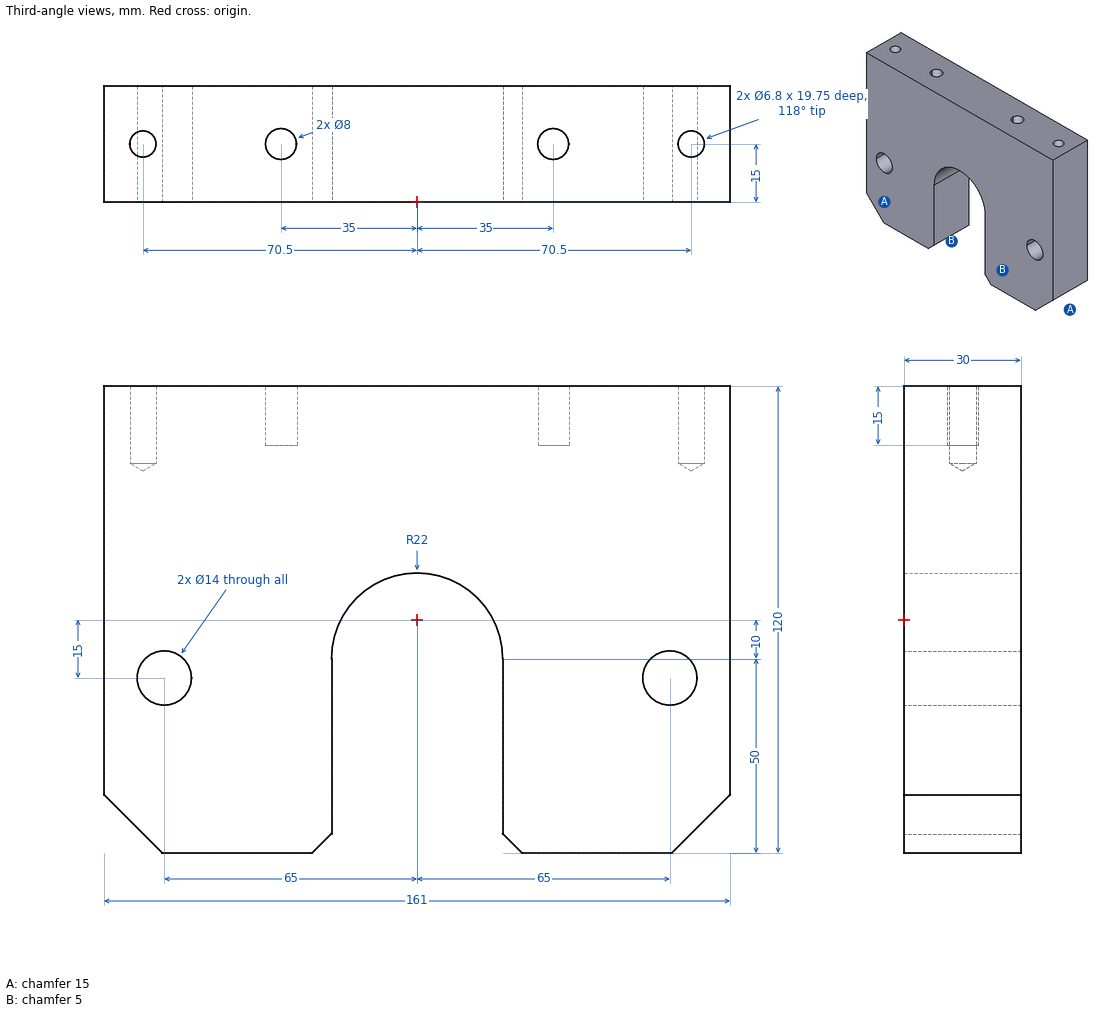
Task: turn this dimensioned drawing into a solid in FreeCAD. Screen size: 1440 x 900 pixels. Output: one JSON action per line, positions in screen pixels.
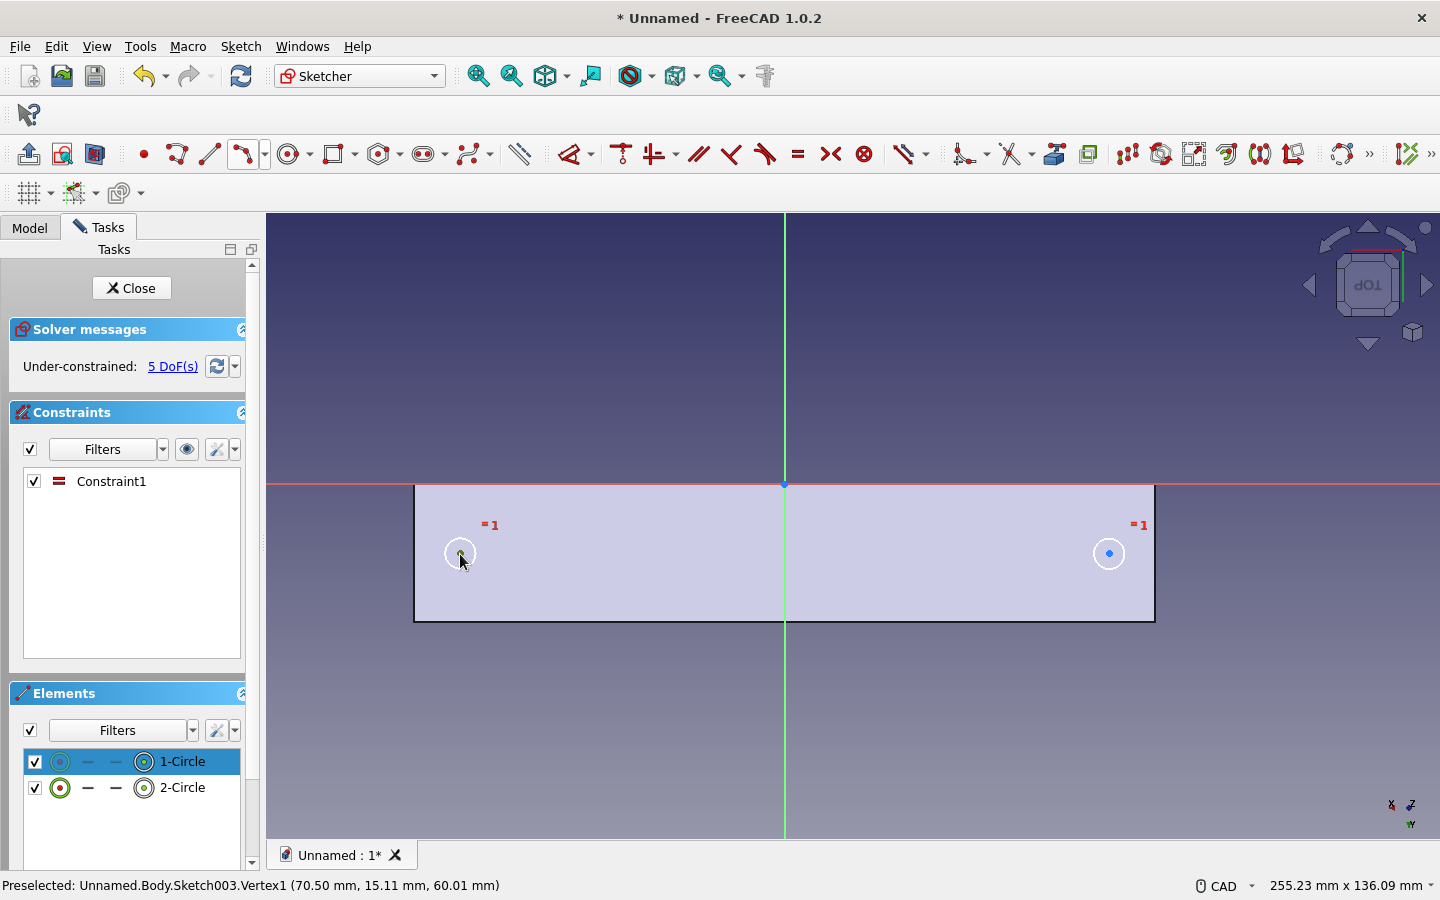
{"action": "left_click", "coordinate": [1109, 554]}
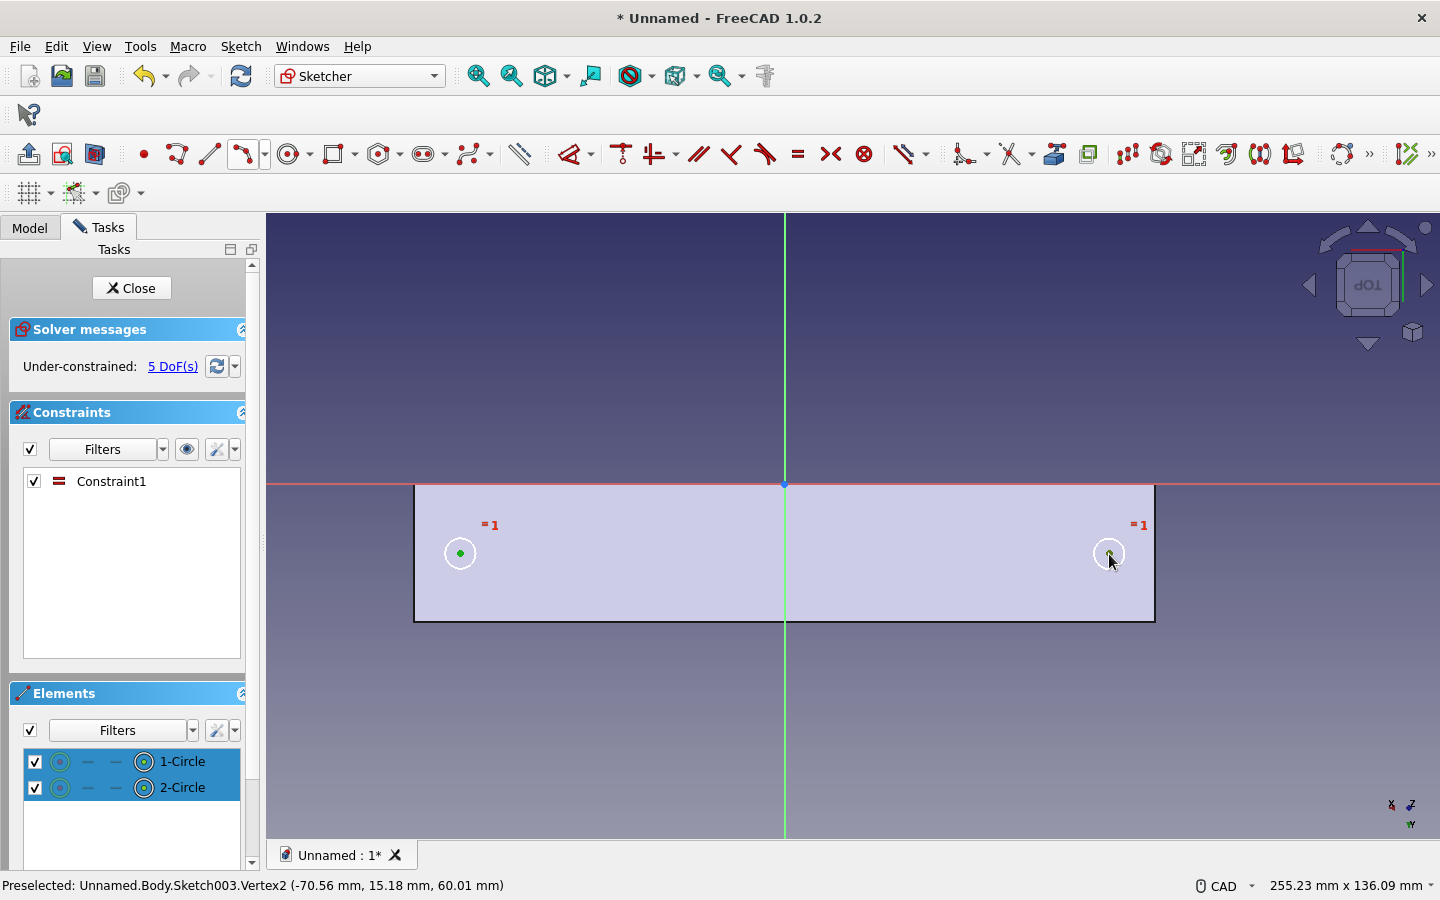
{"action": "key", "text": "h"}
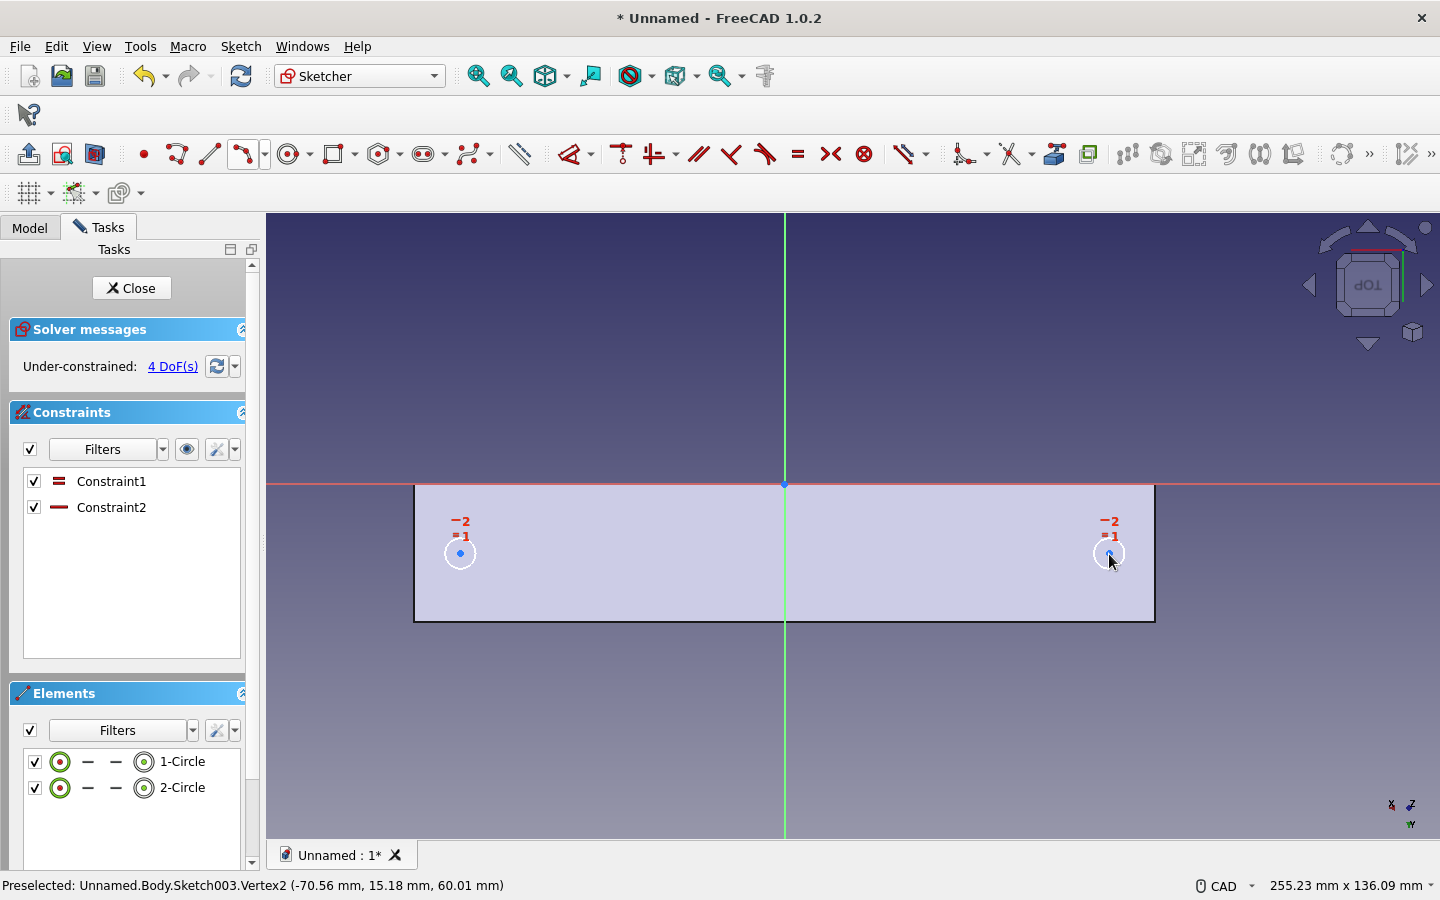
{"action": "key", "text": "d"}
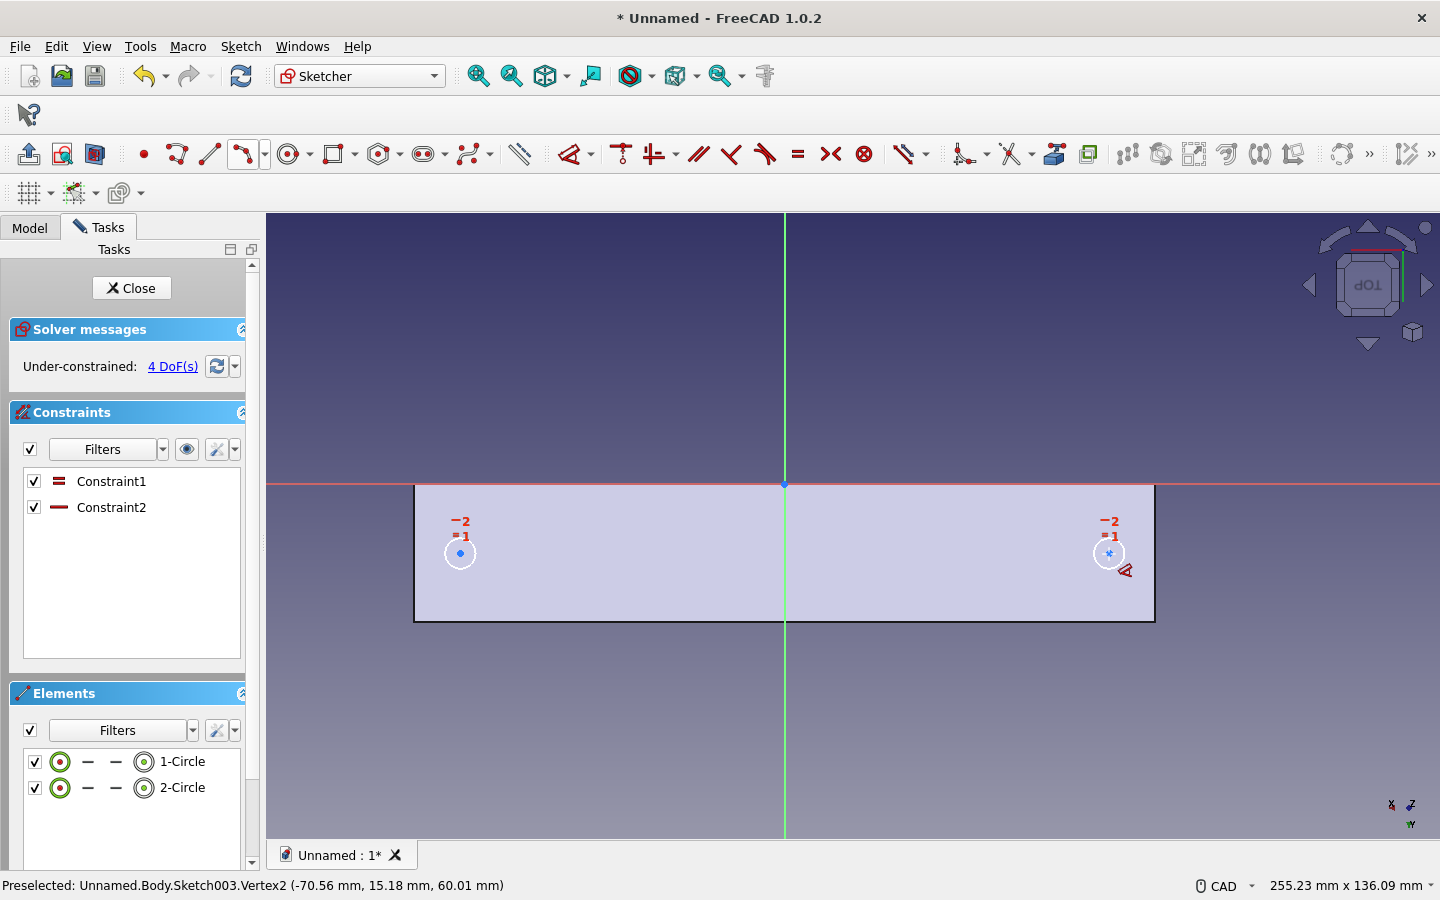
{"action": "scroll", "coordinate": [471, 543], "scroll_direction": "up", "scroll_amount": 2}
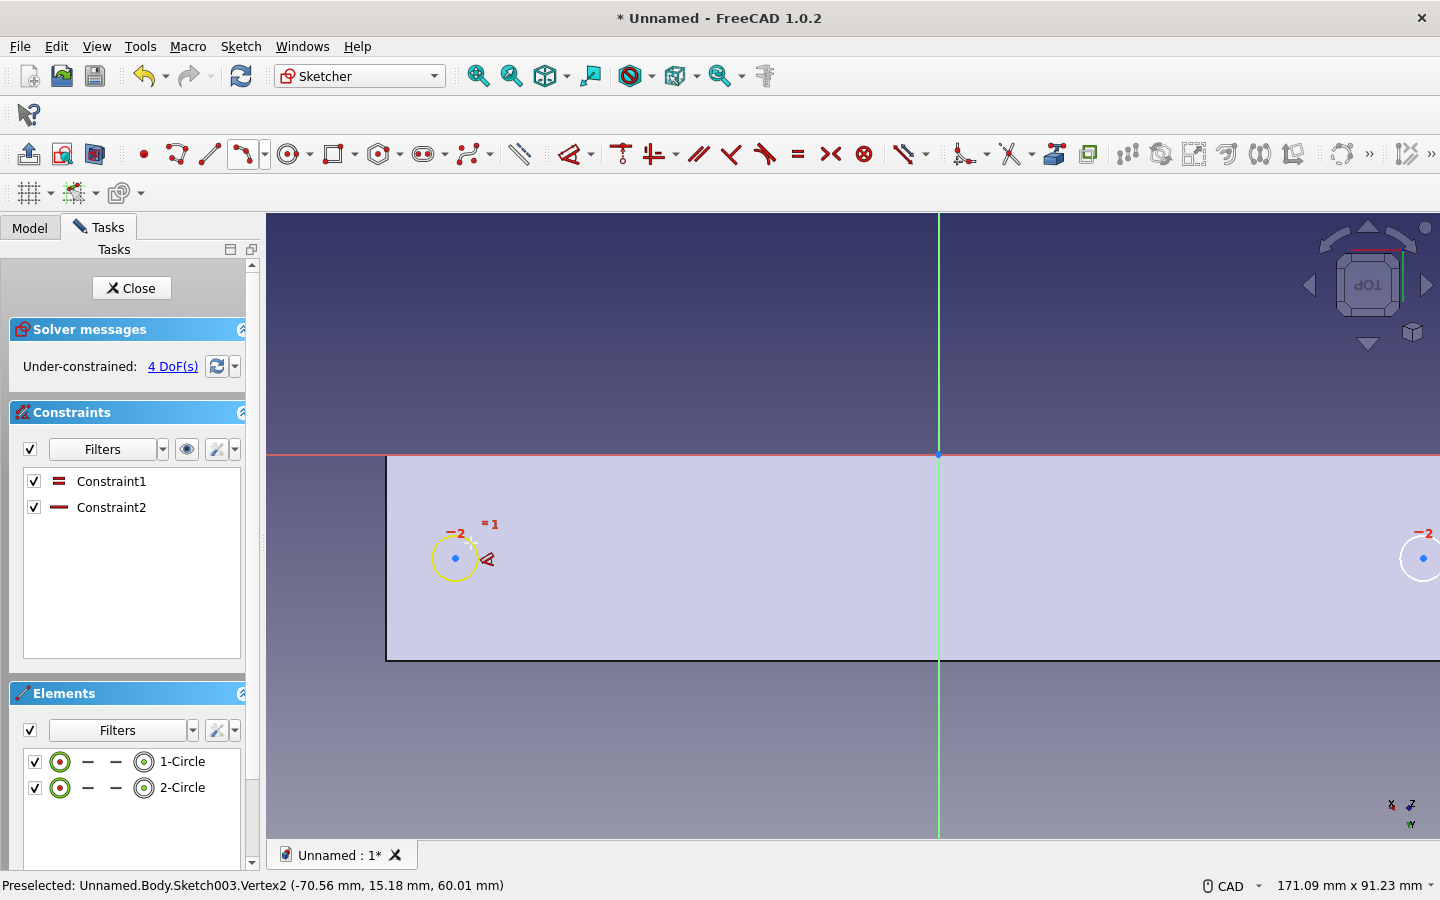
{"action": "left_click", "coordinate": [471, 542]}
{"action": "left_click", "coordinate": [493, 519]}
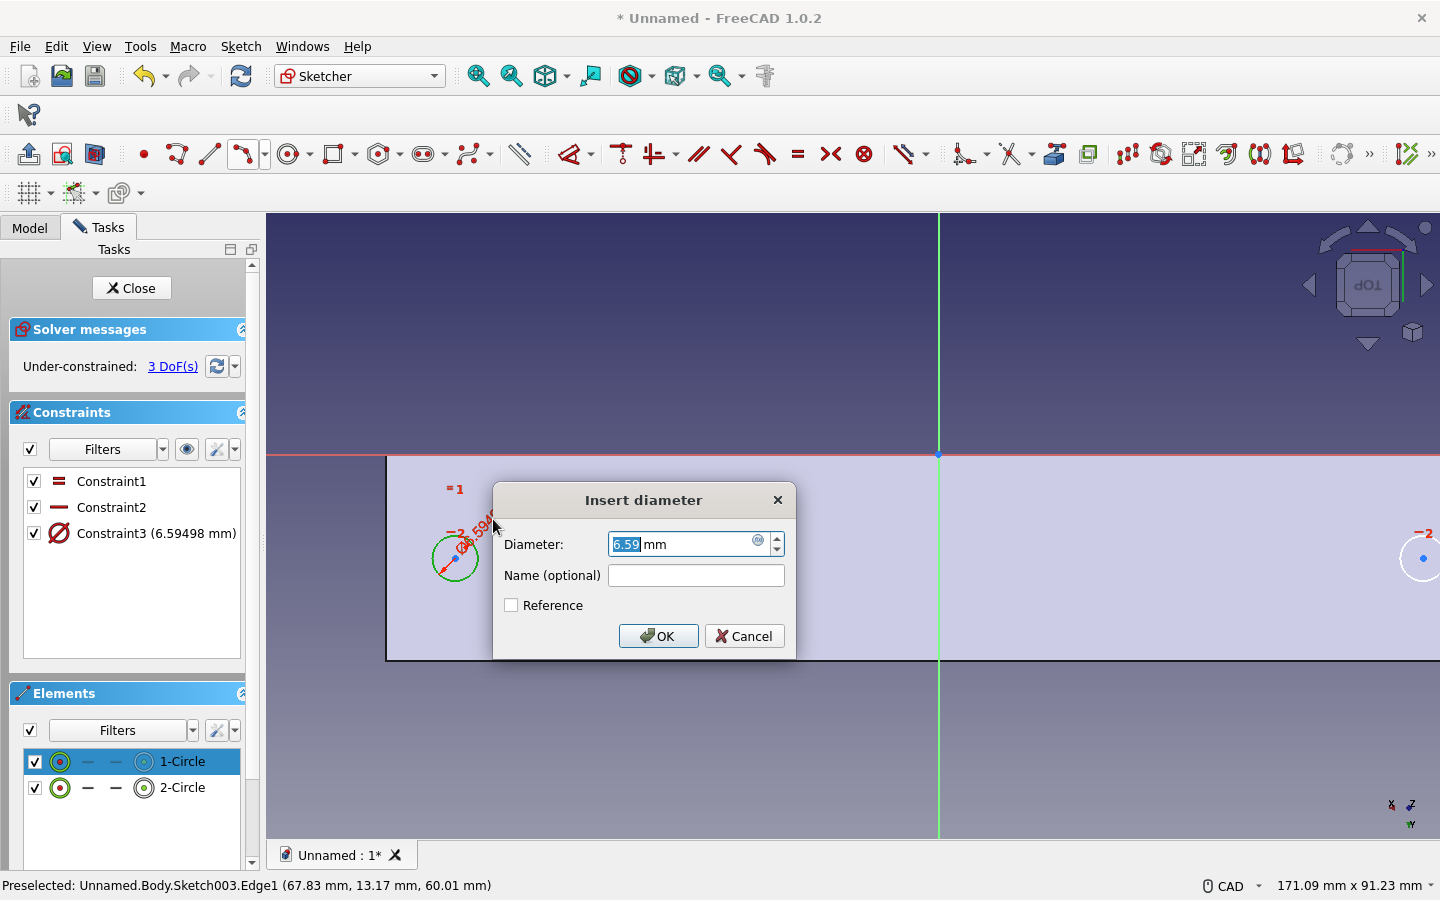
{"action": "type", "text": "6.8"}
{"action": "key", "text": "Return"}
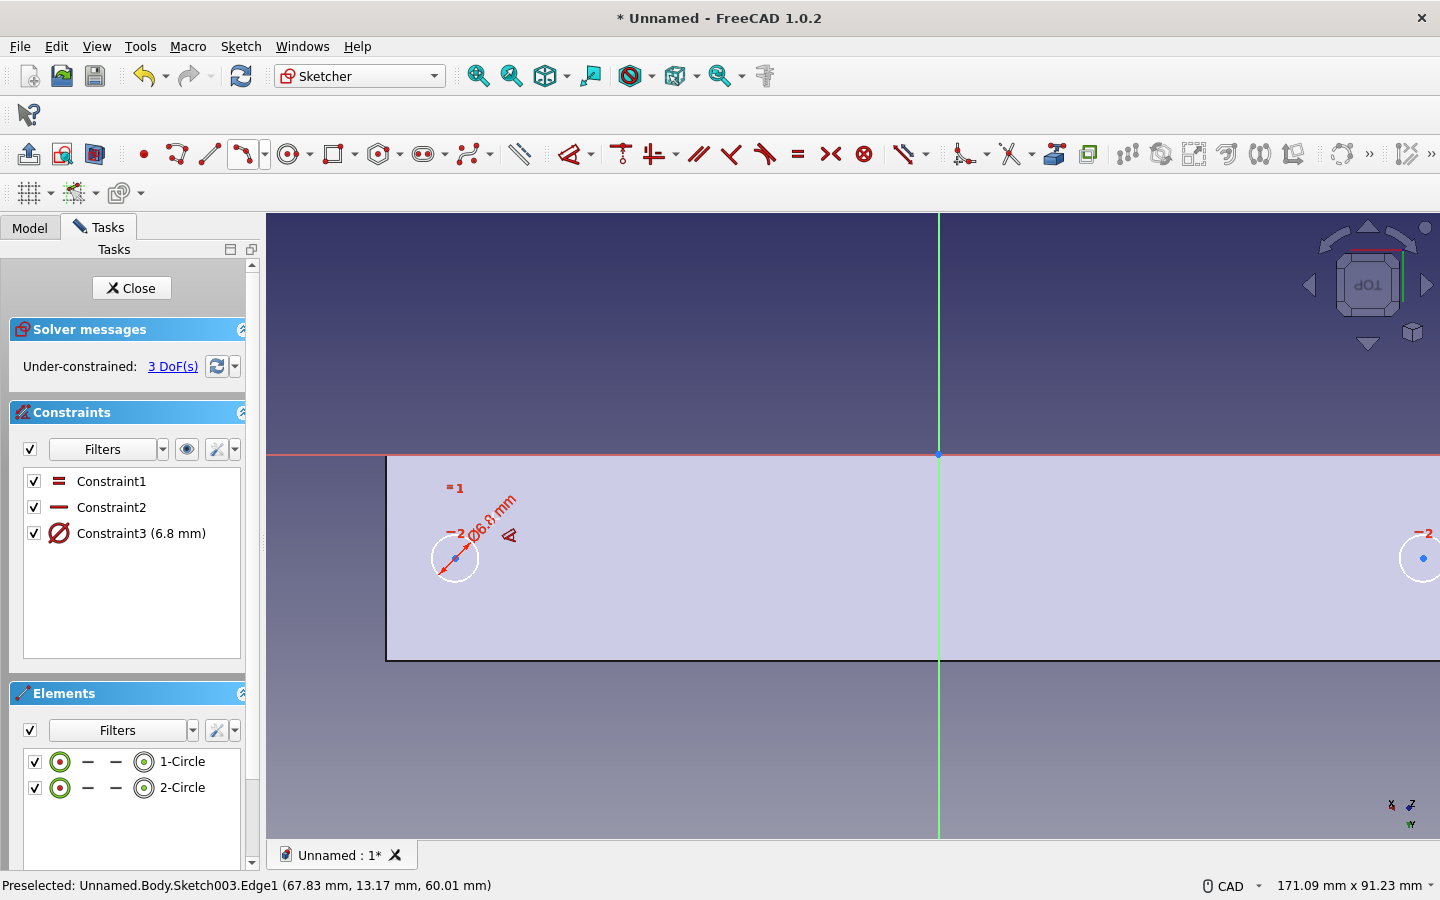
{"action": "left_click", "coordinate": [455, 558]}
{"action": "left_click", "coordinate": [421, 507]}